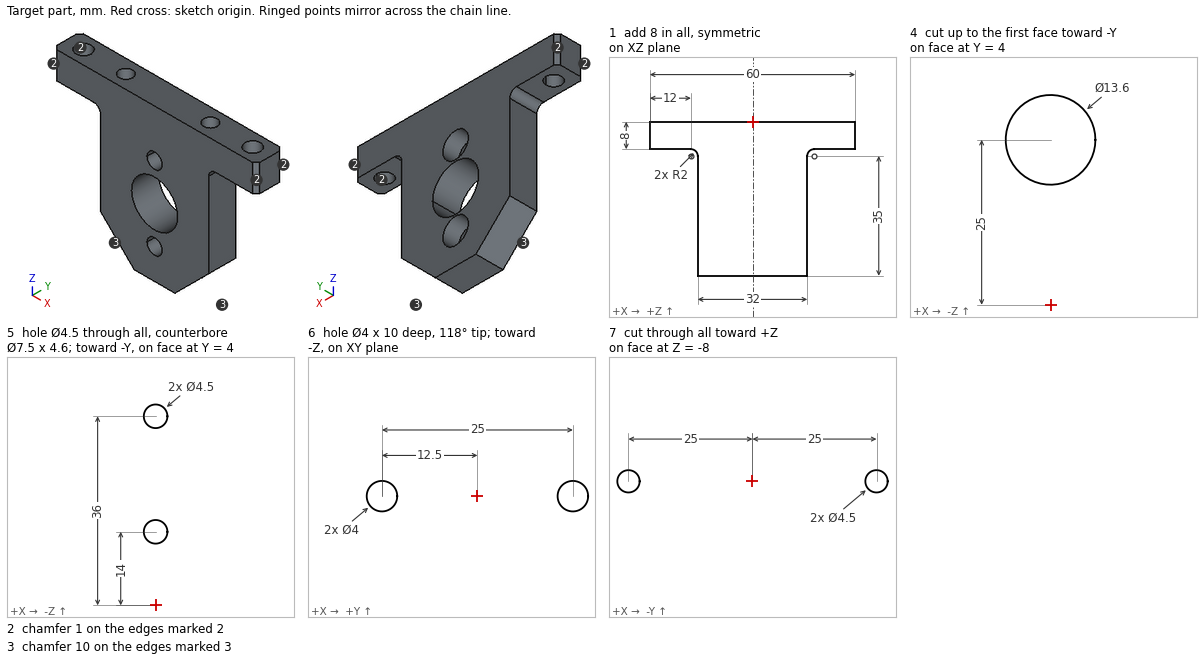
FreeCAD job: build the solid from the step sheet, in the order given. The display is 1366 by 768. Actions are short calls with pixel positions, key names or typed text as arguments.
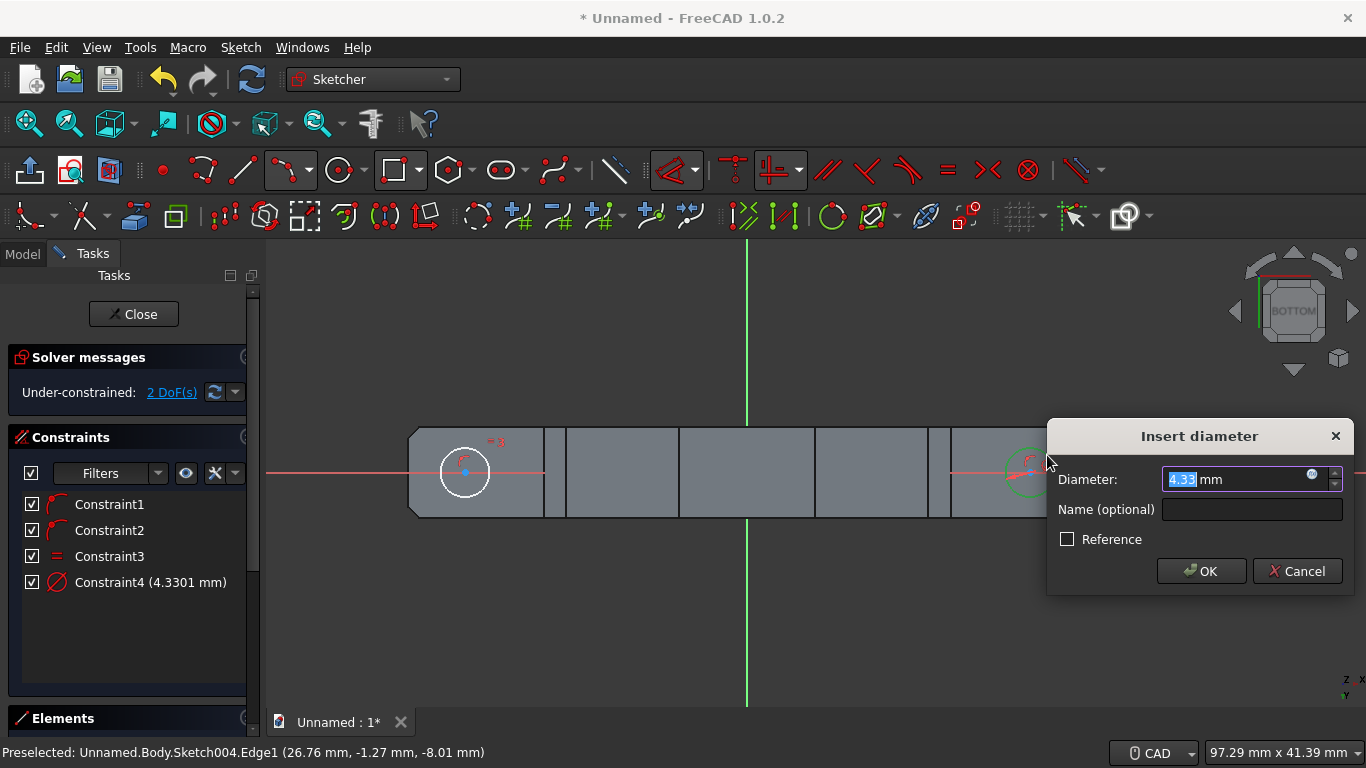
text(4.5)
key(Return)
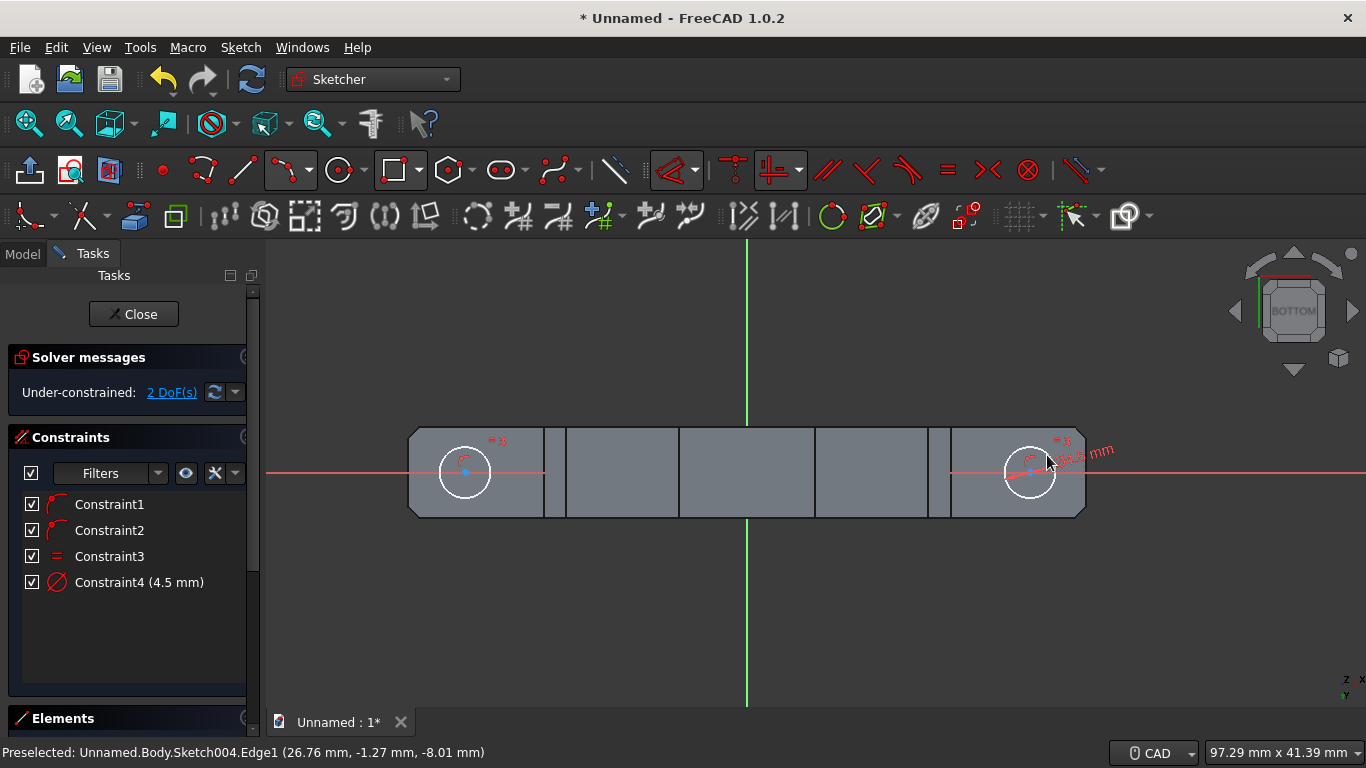
click(1030, 473)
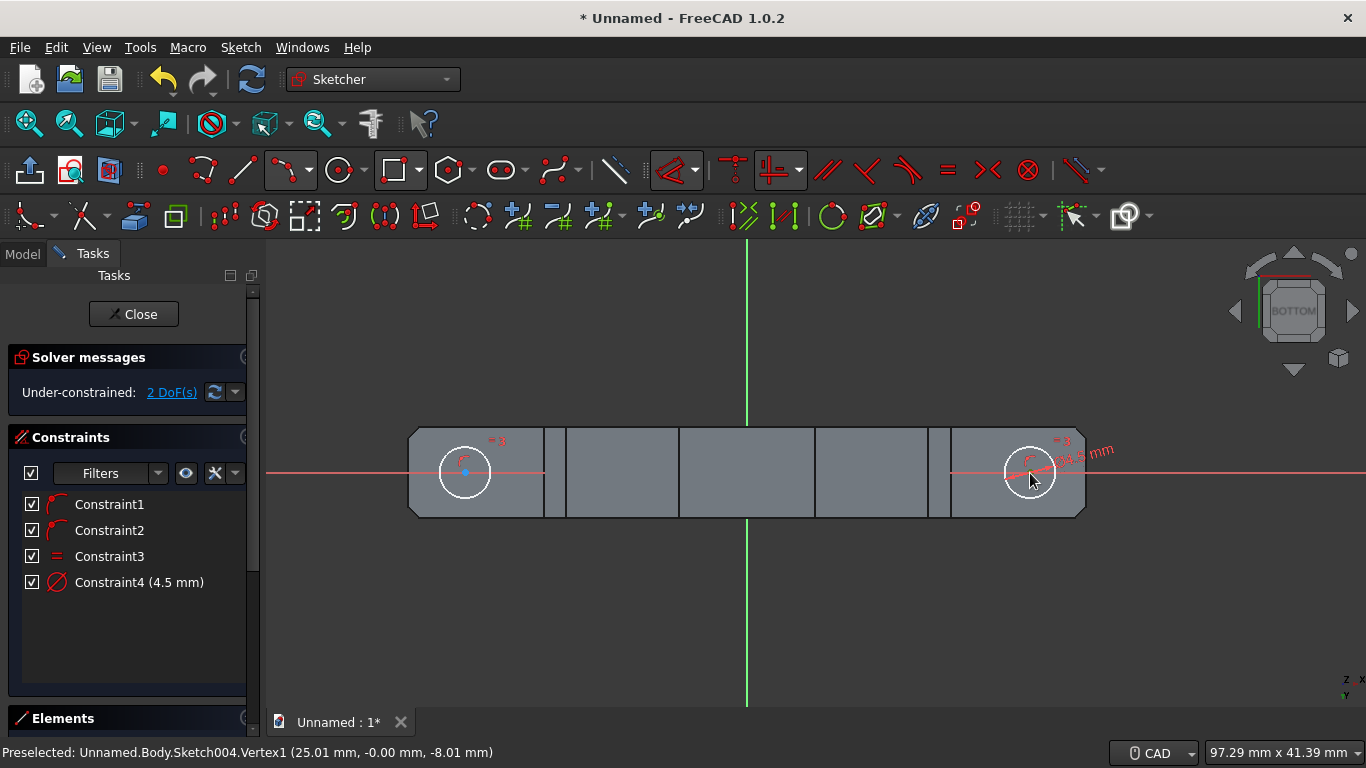
key(l)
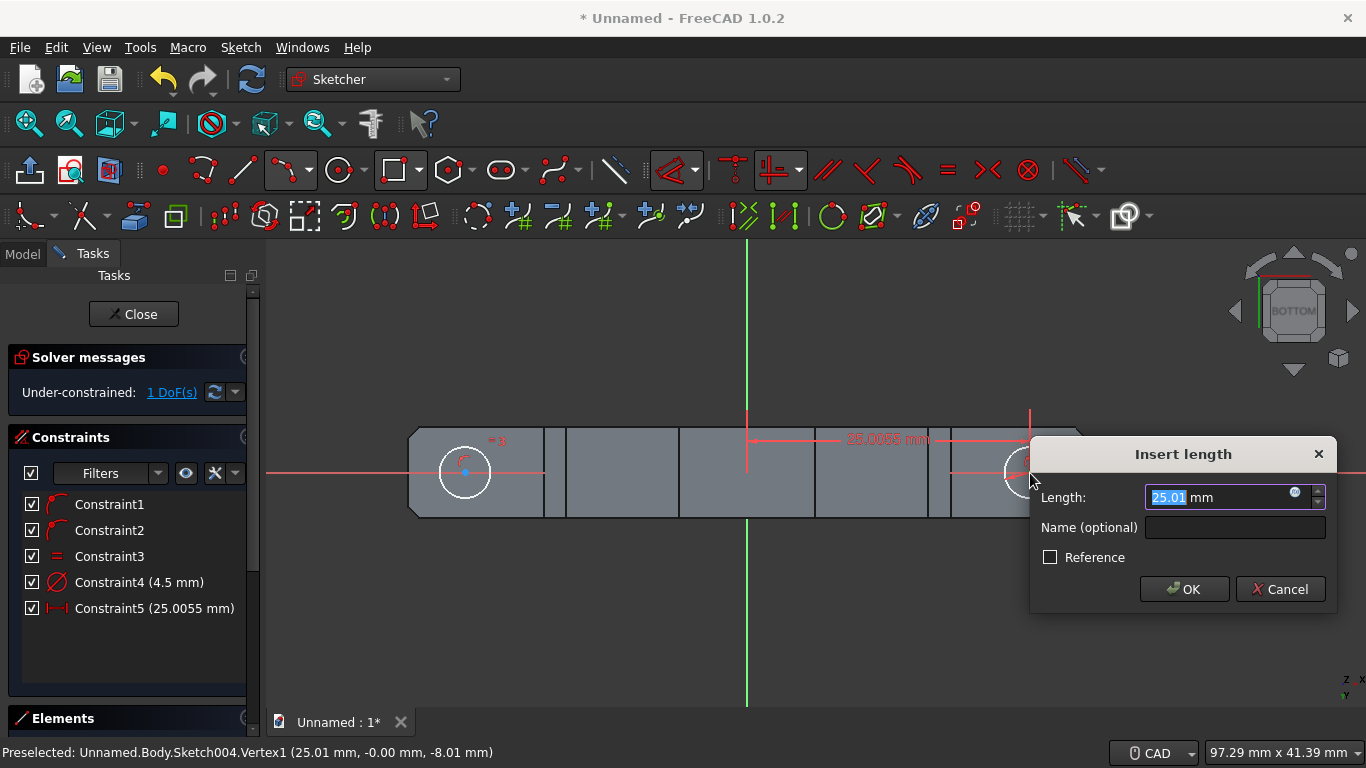
text(25)
key(Return)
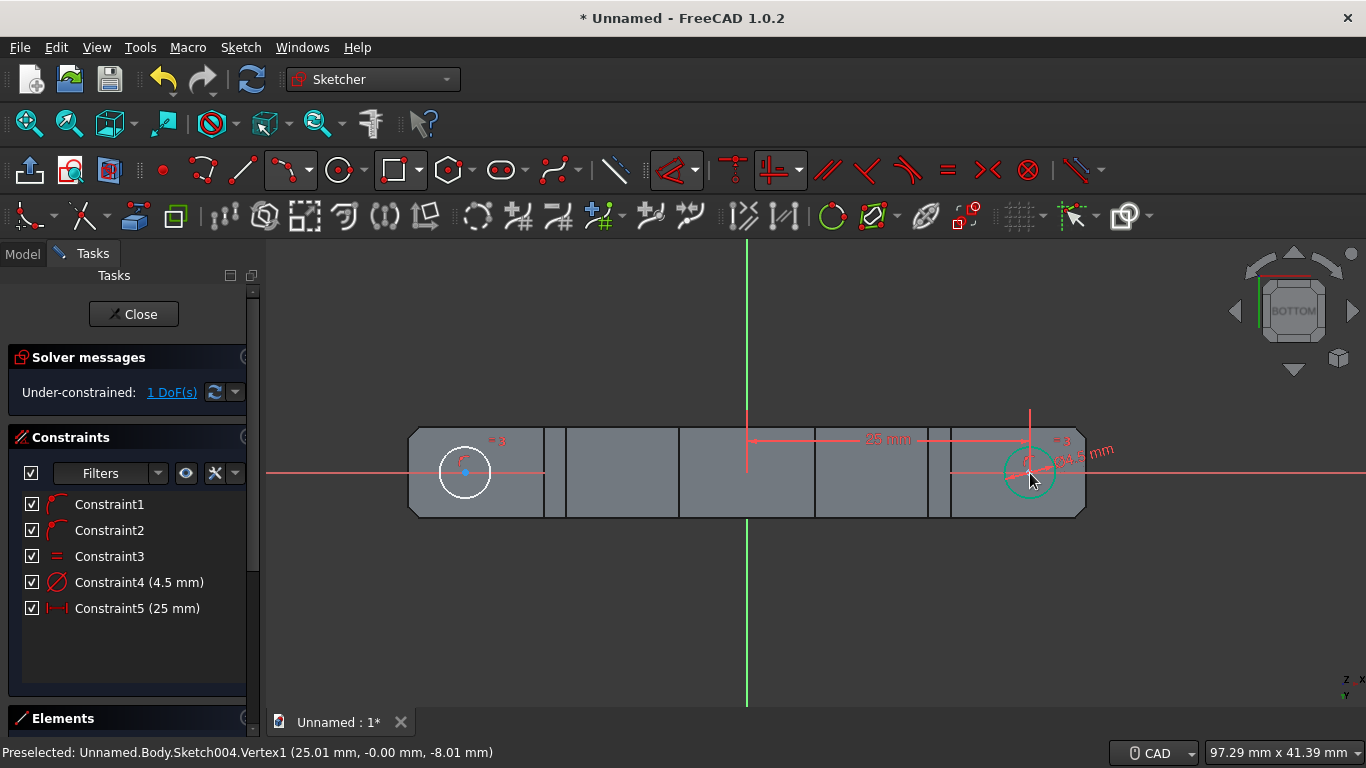
click(465, 473)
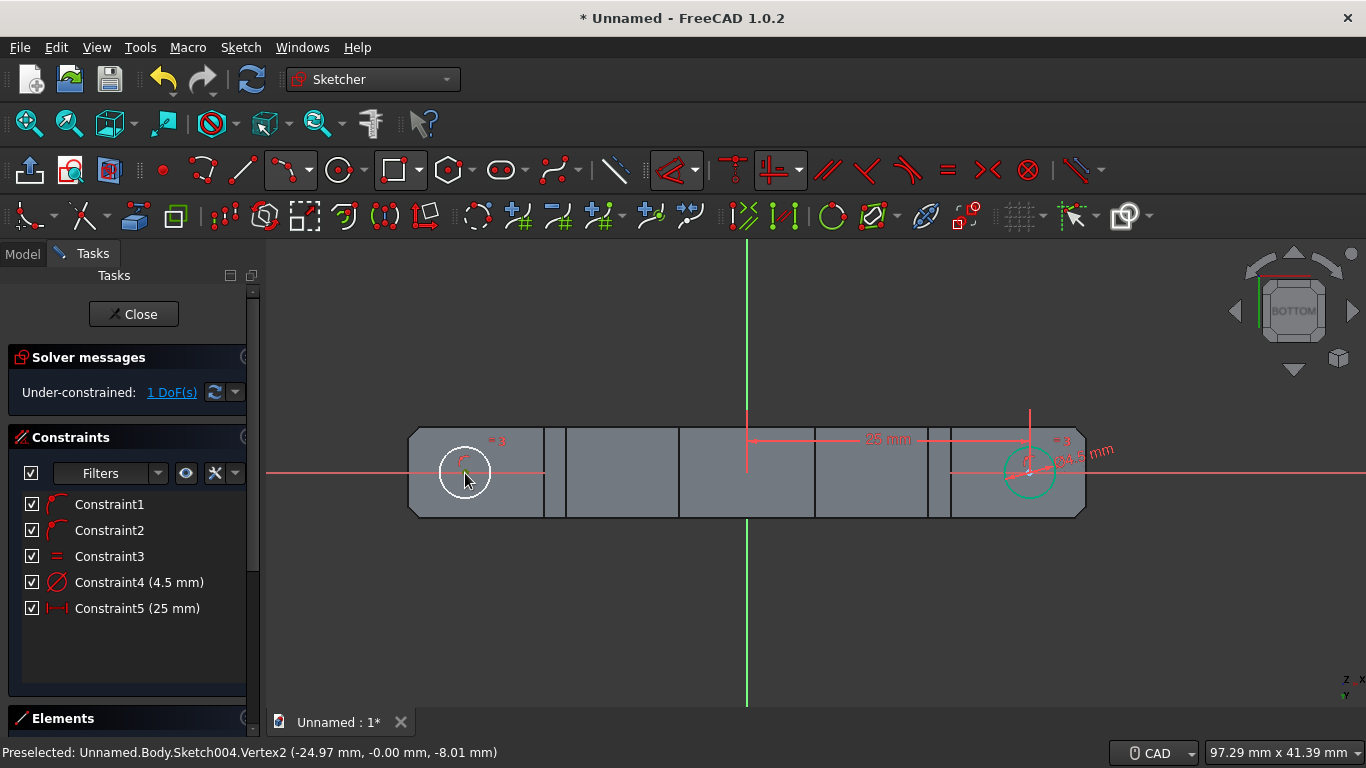
key(l)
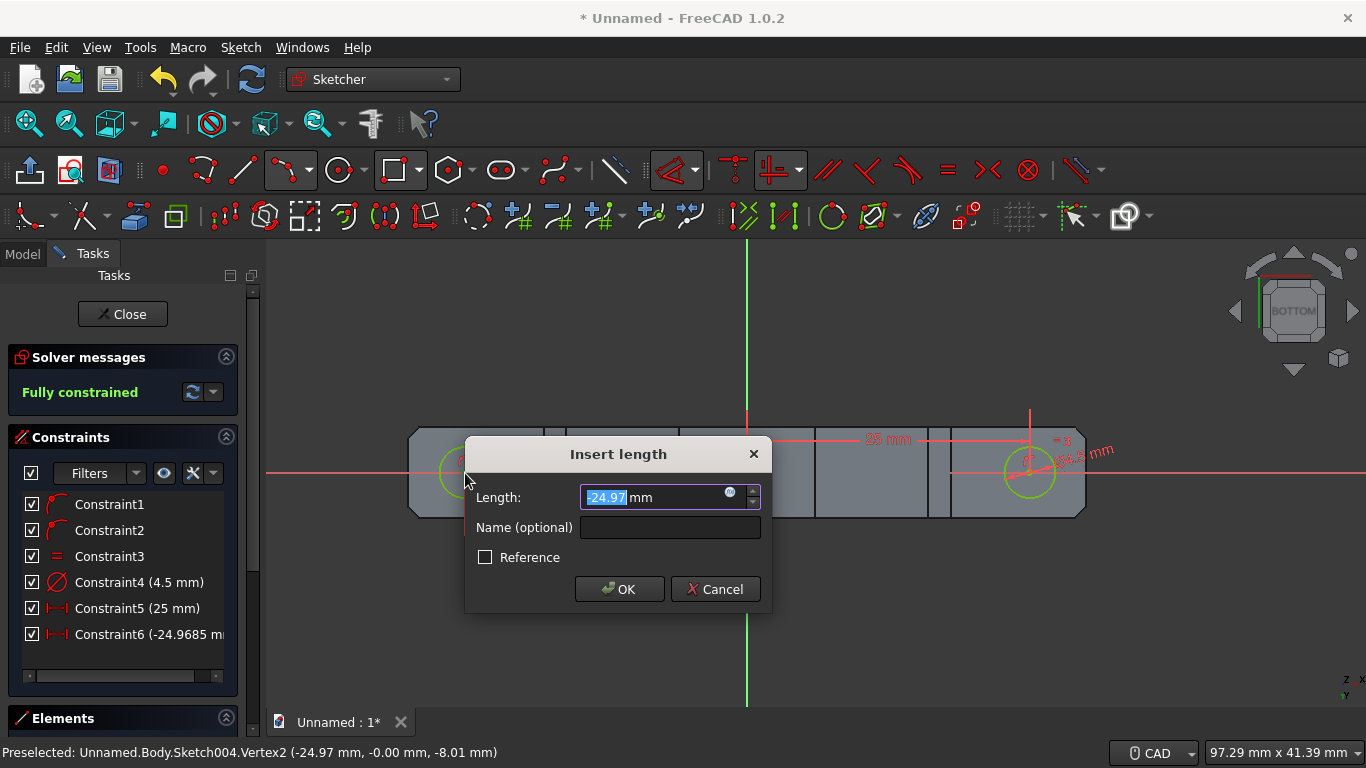
text(-25)
key(Return)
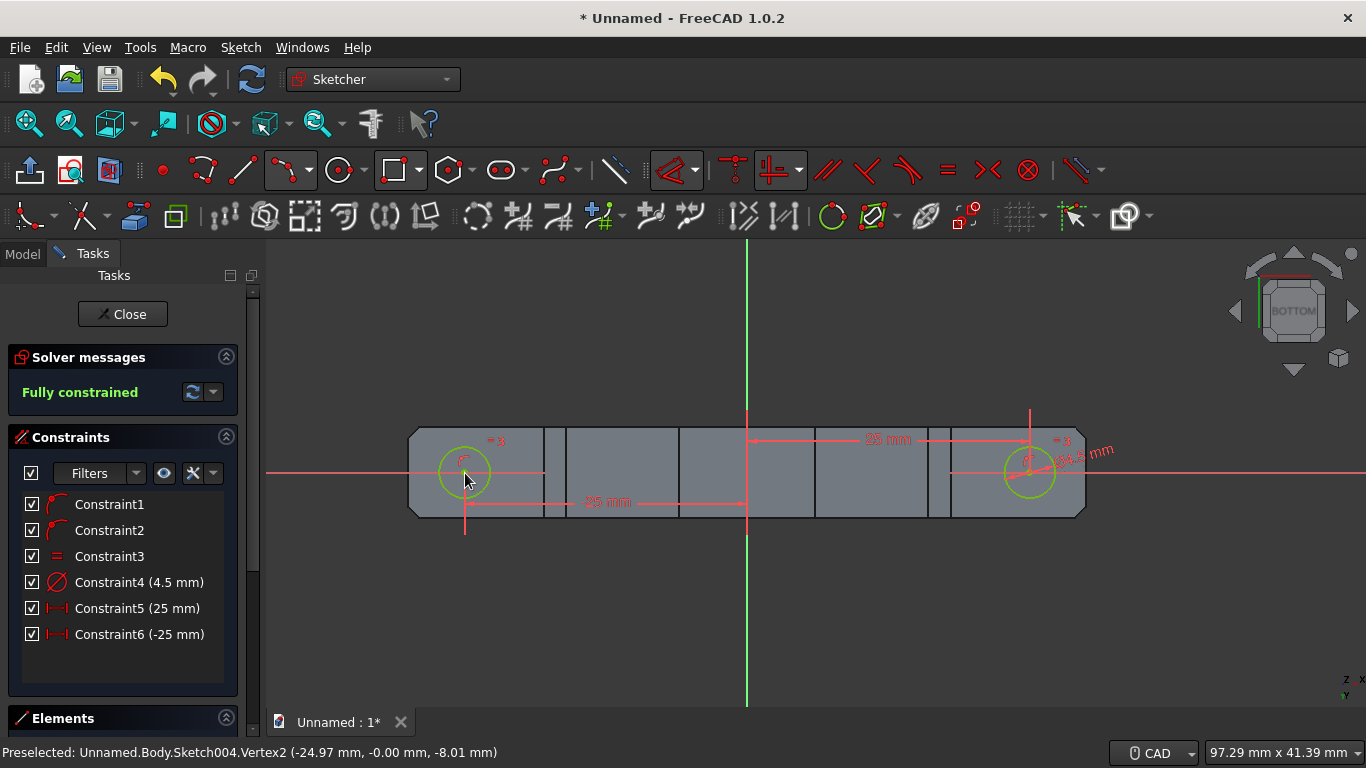
click(123, 314)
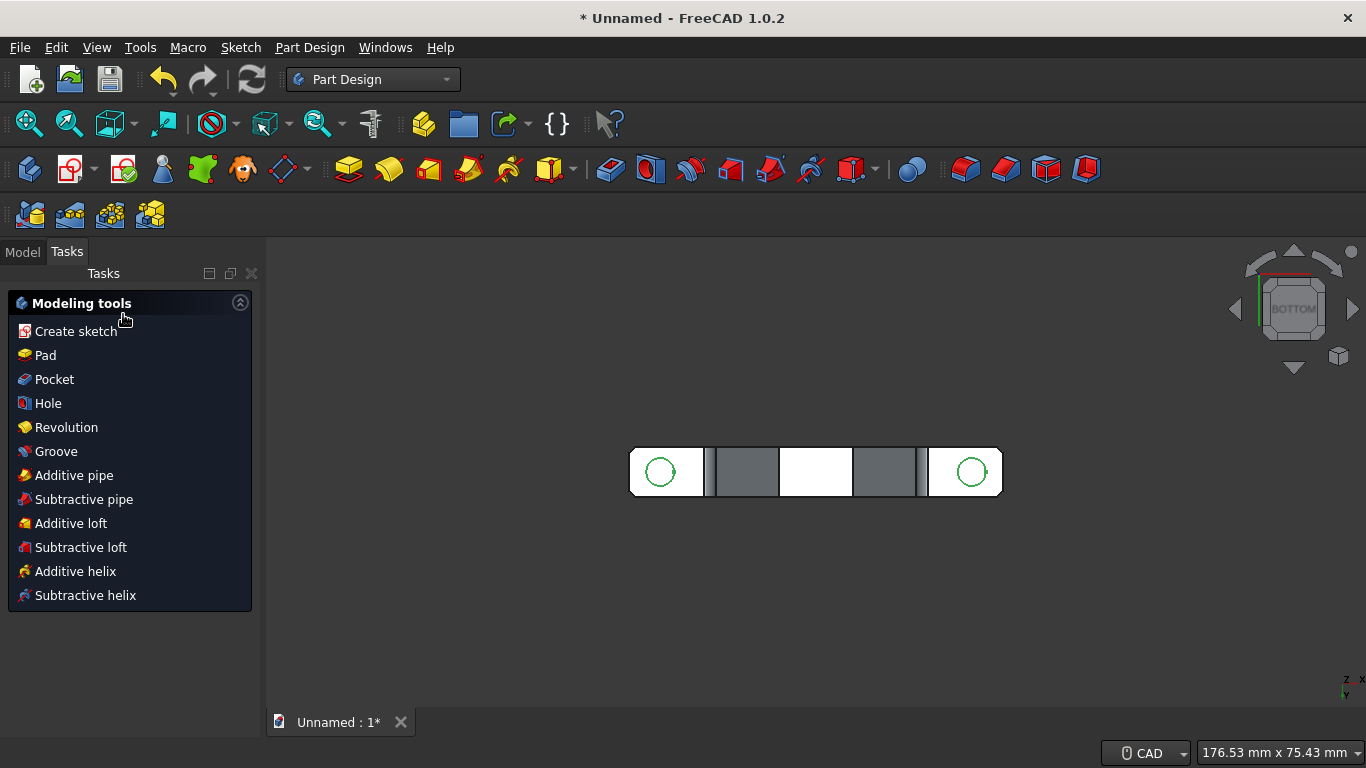
click(612, 170)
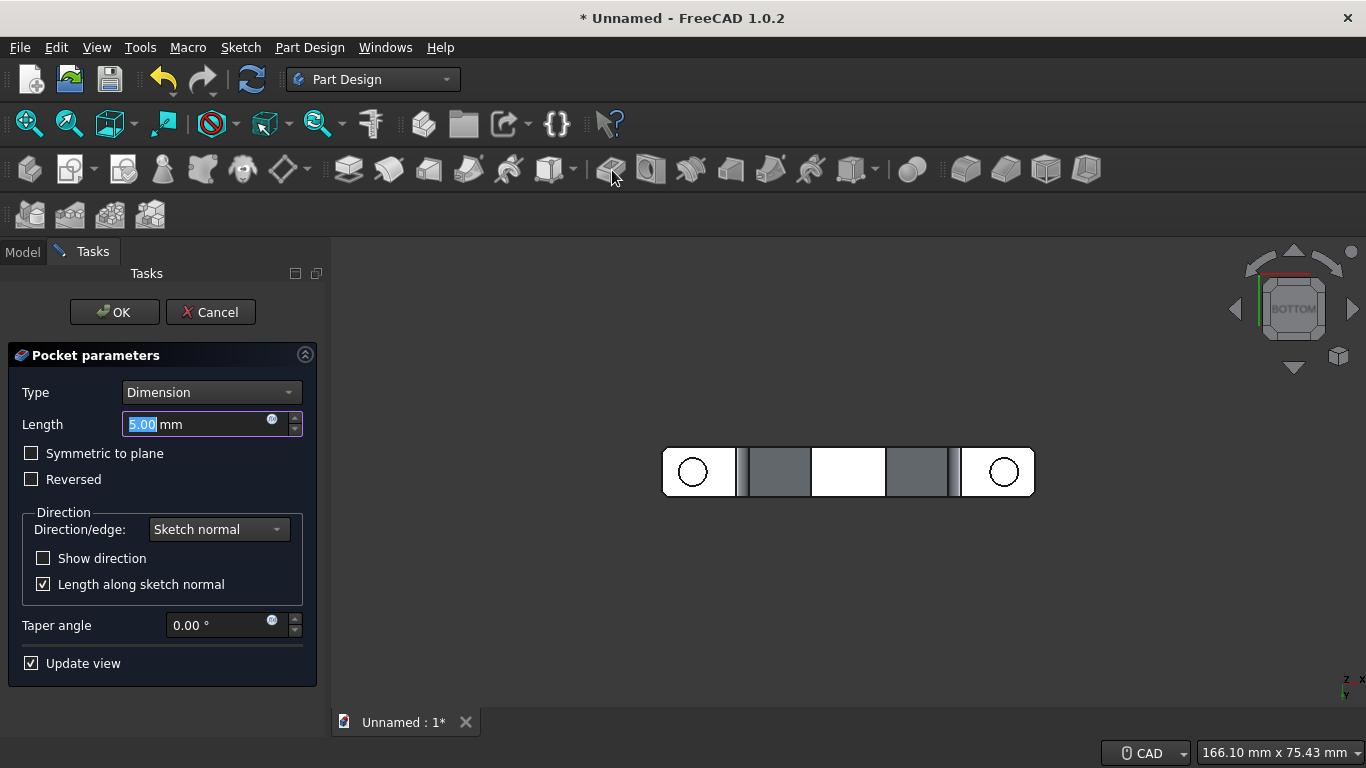
click(212, 392)